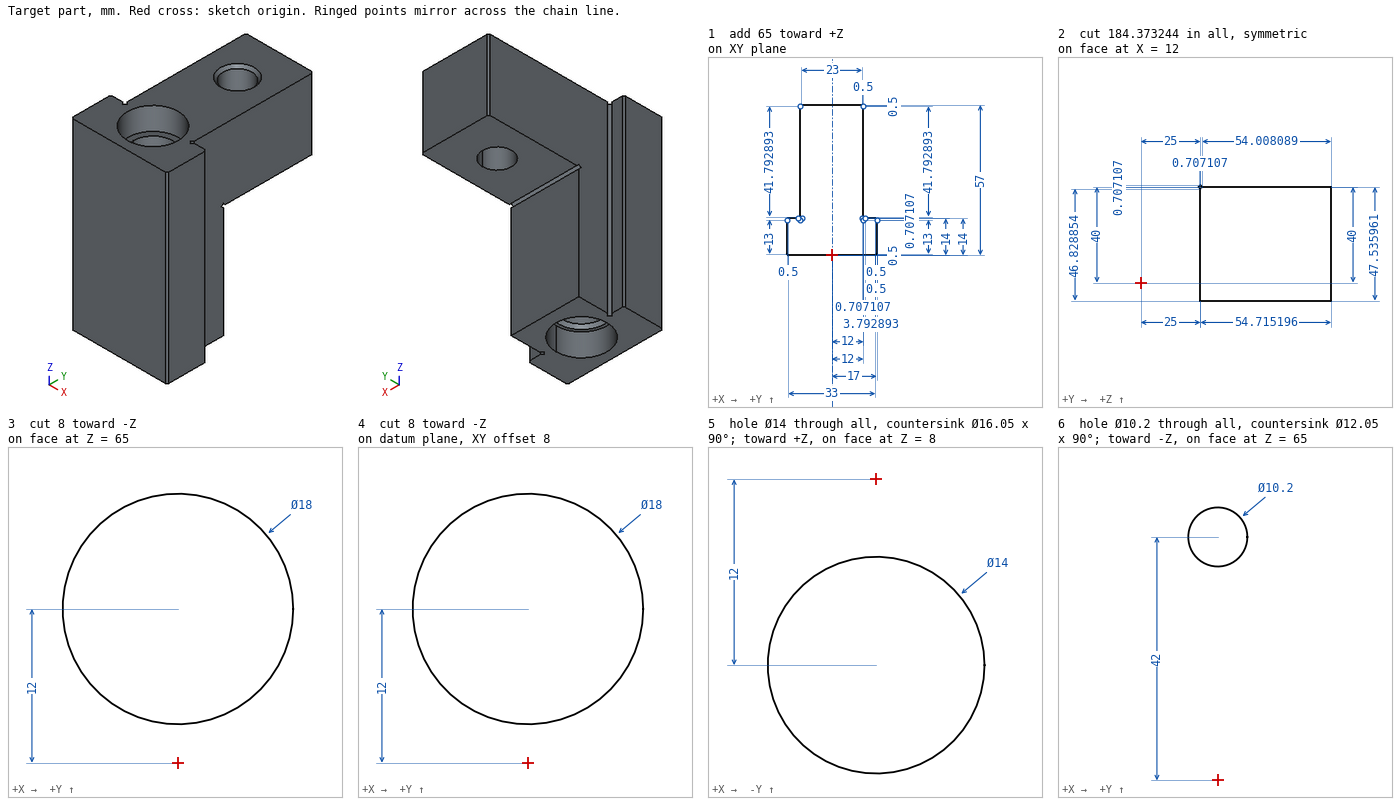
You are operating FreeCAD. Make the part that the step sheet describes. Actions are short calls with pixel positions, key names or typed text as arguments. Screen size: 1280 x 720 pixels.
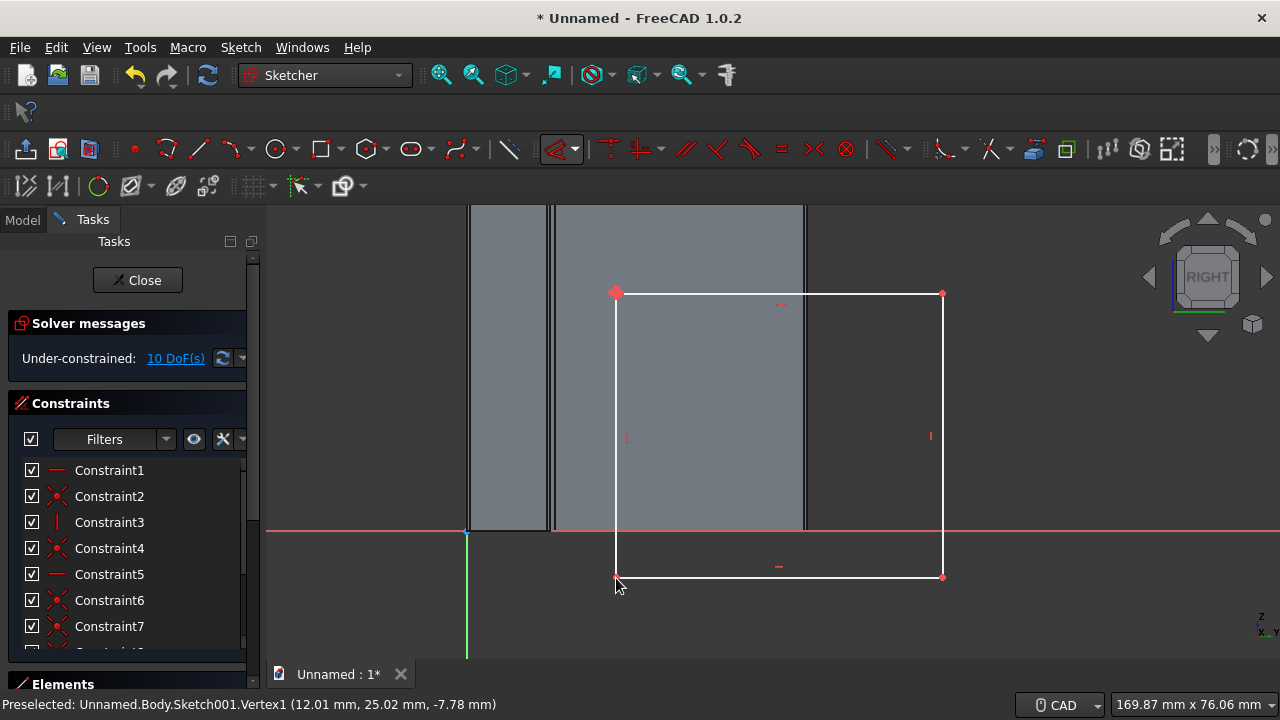
key(d)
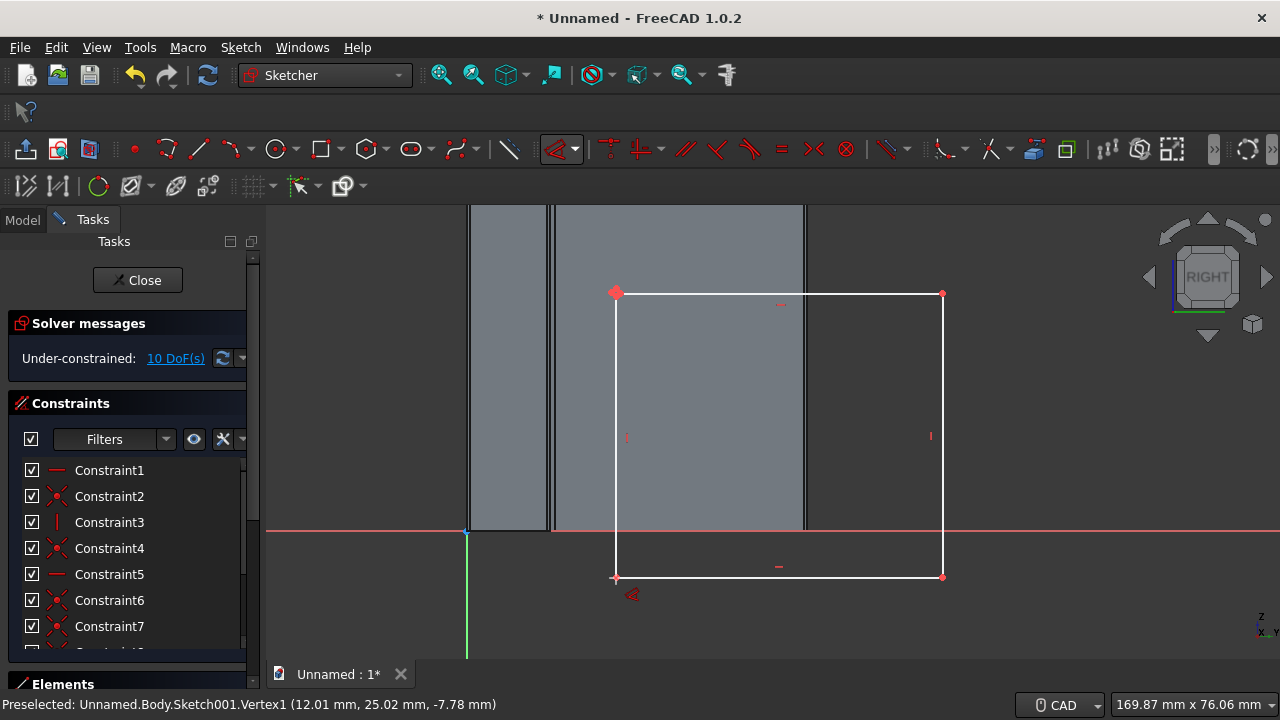
click(616, 578)
click(542, 612)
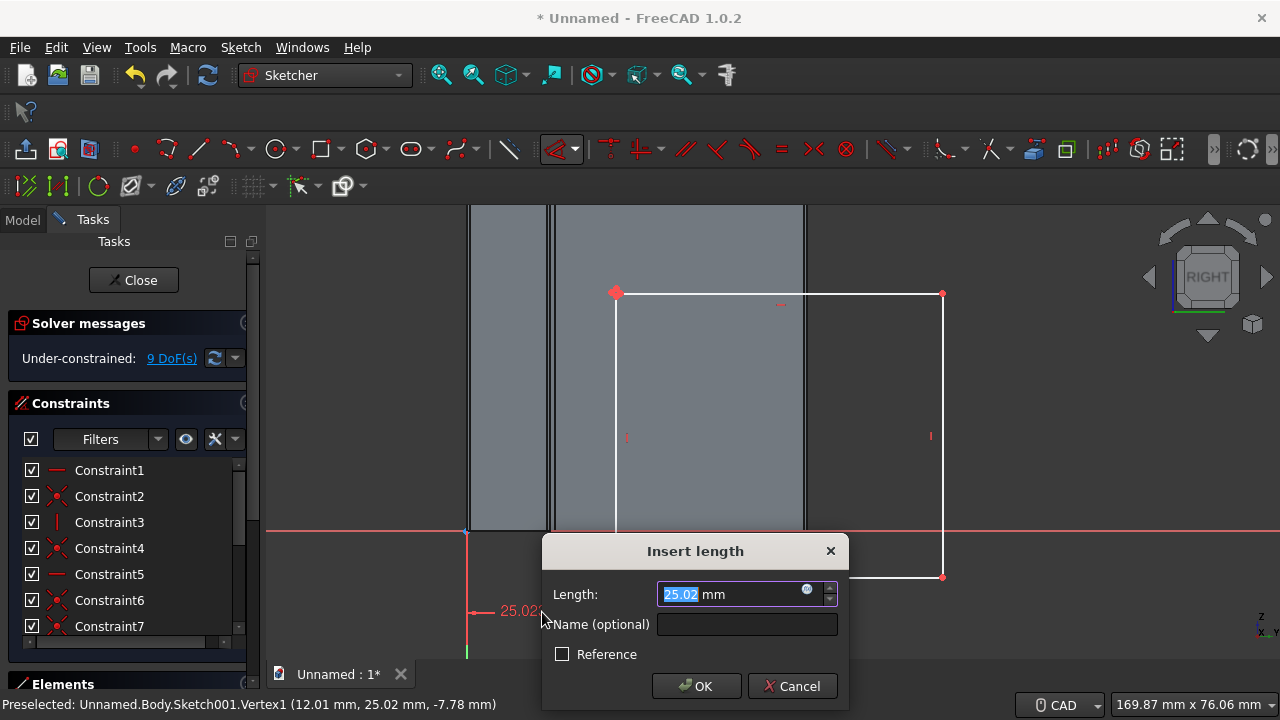
text(25)
key(Return)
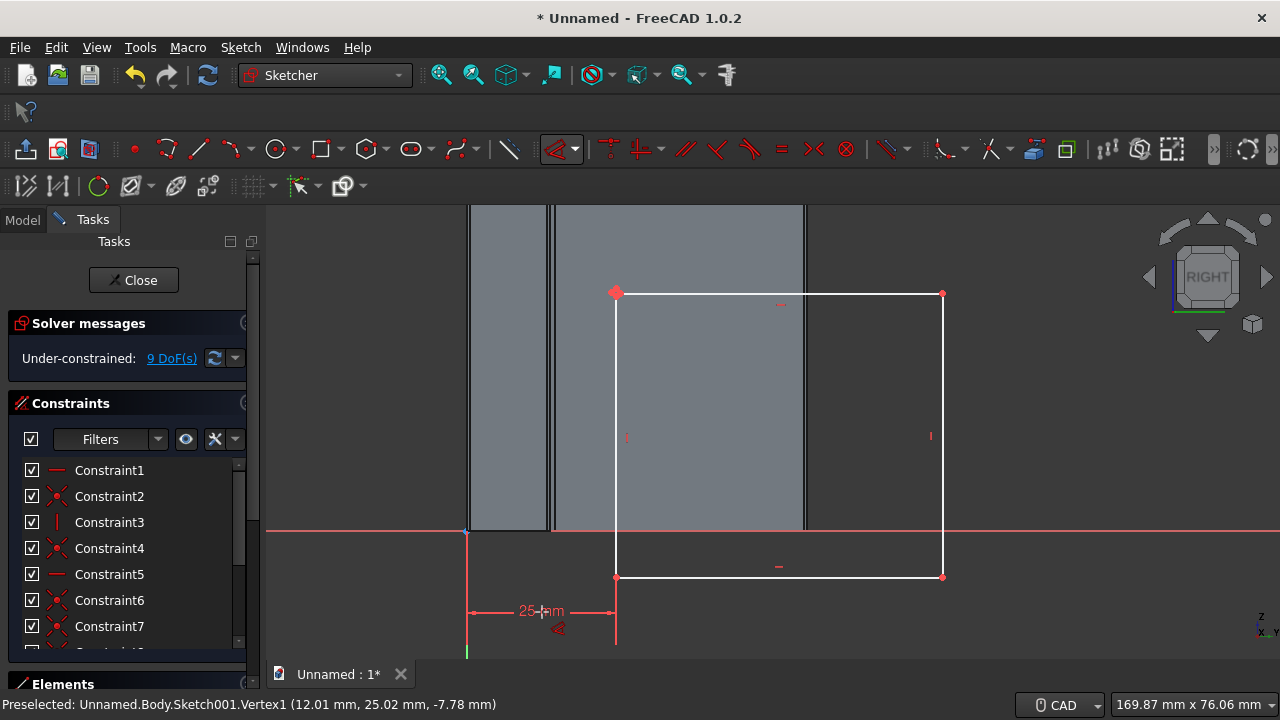
click(943, 294)
click(433, 412)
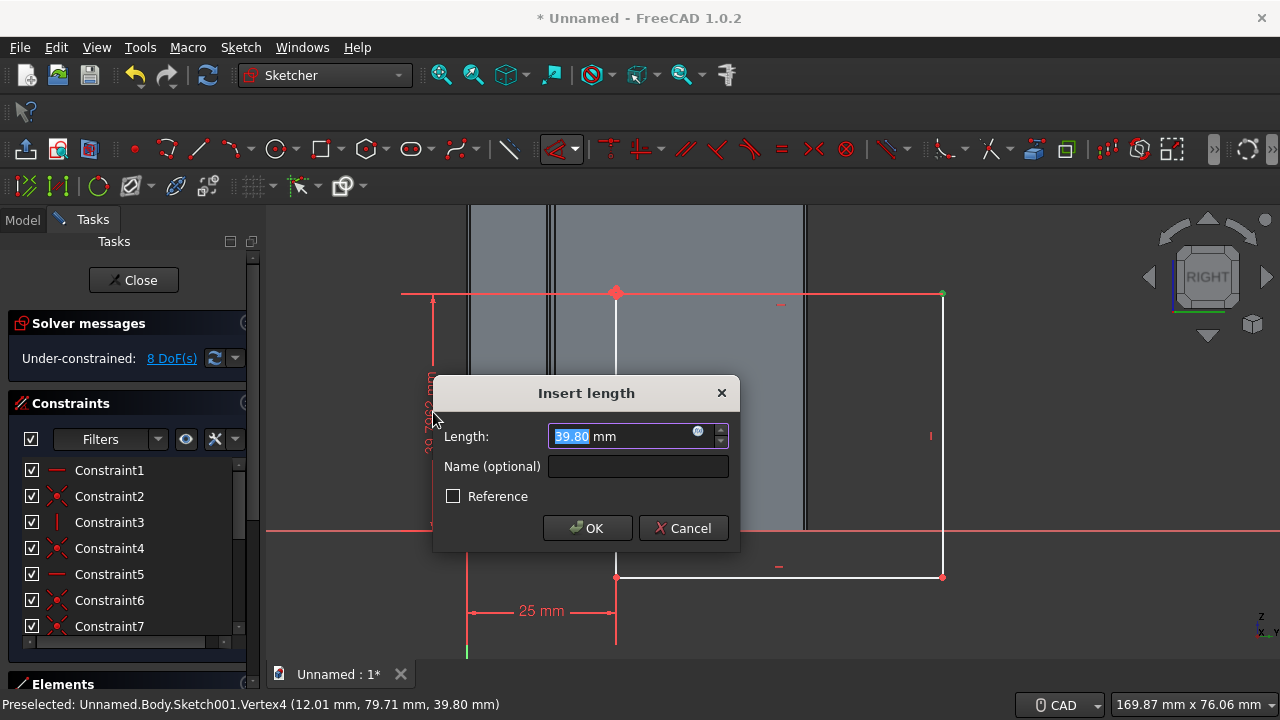
text(40)
key(Return)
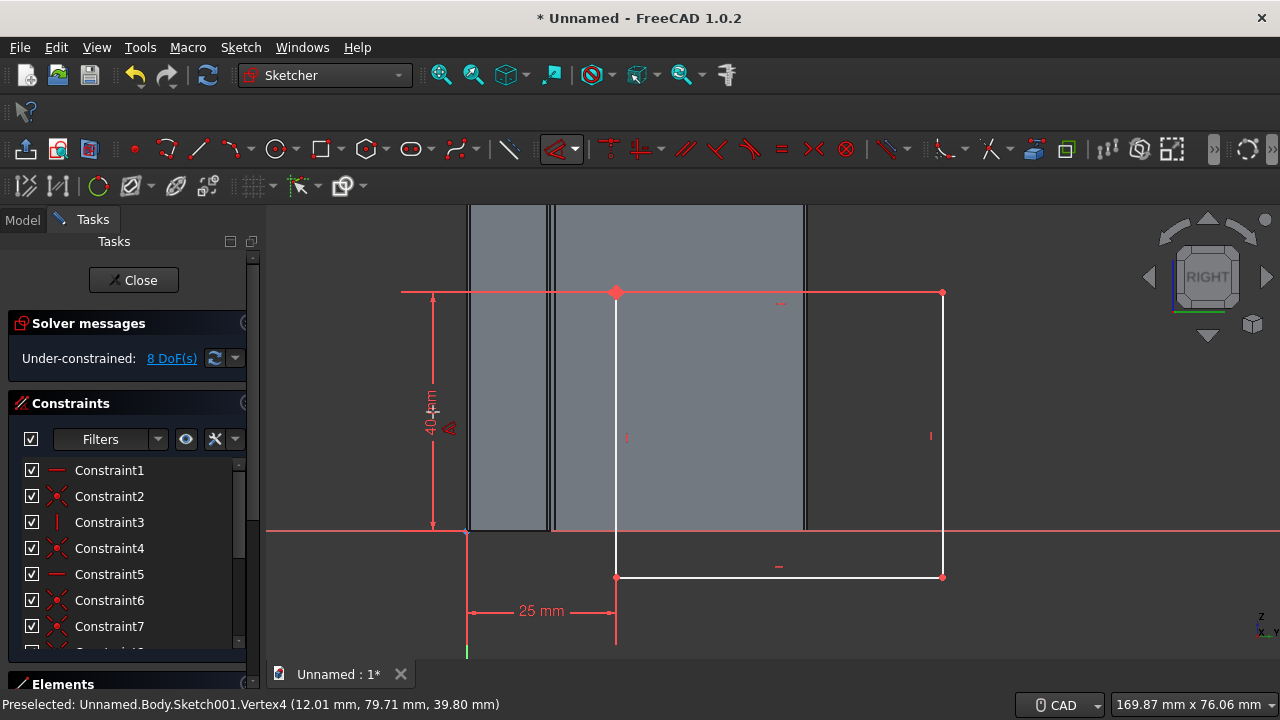
scroll(616, 288, up, 4)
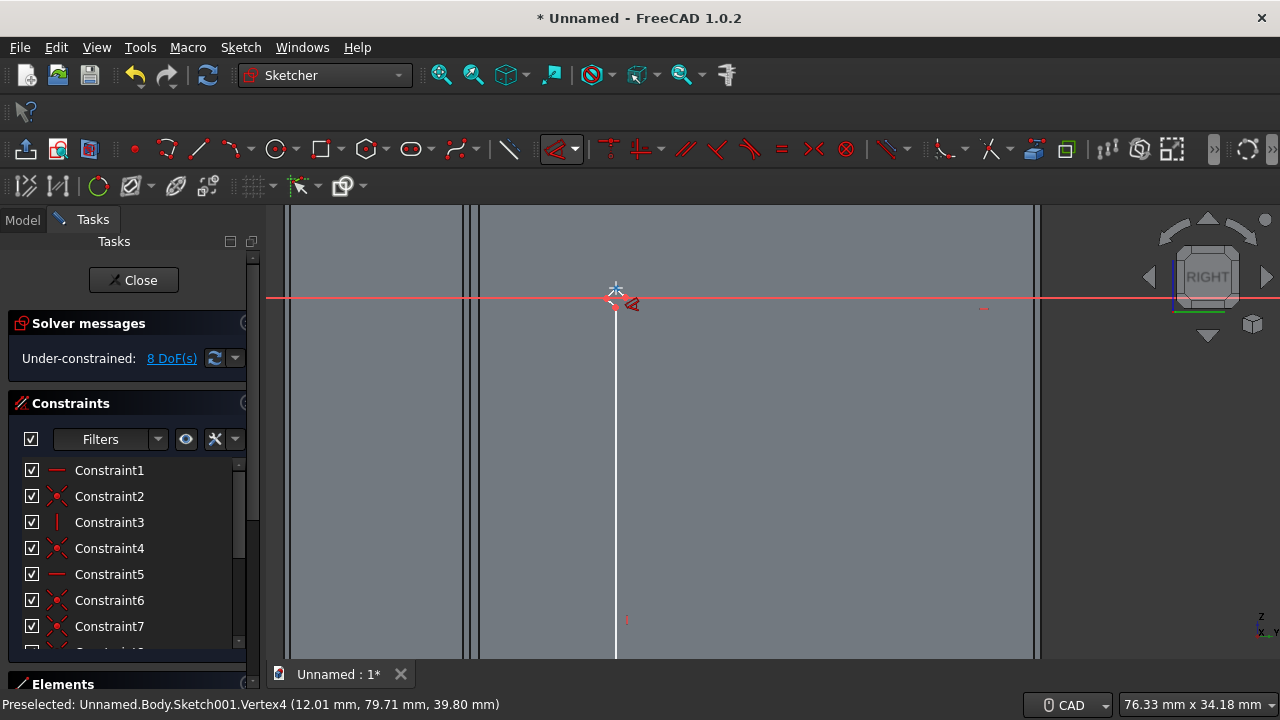
click(616, 289)
click(455, 255)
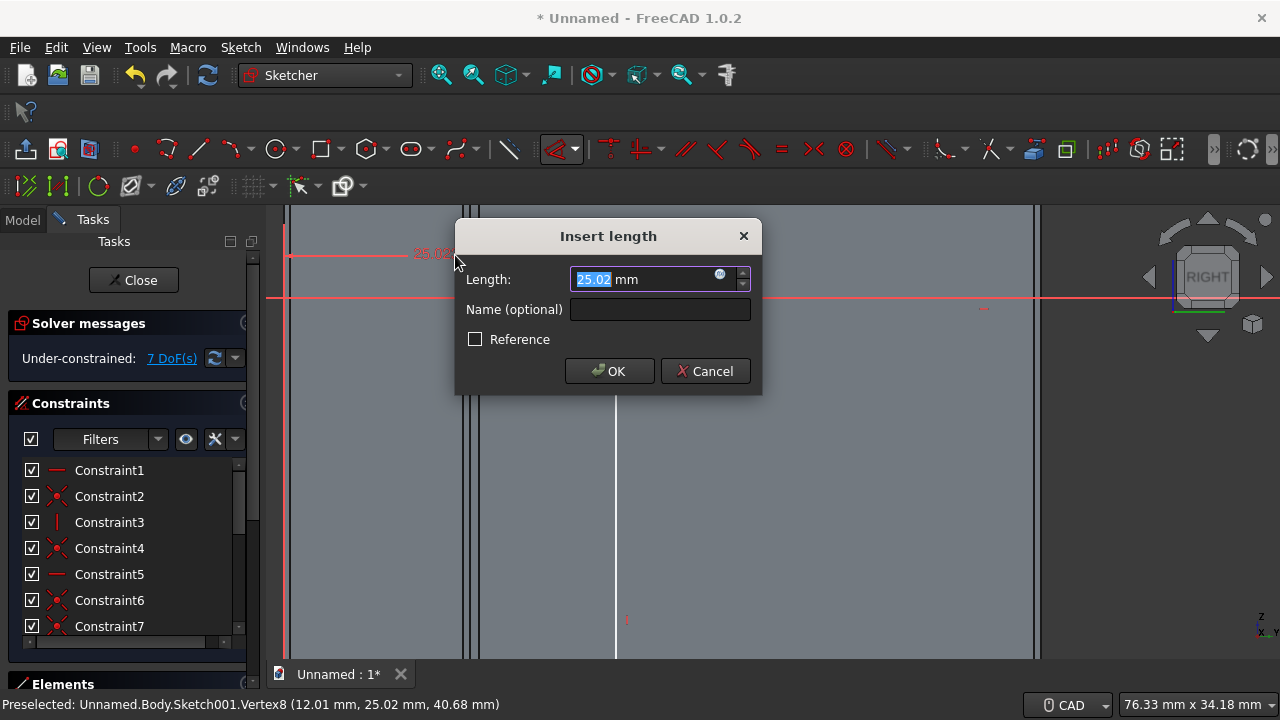
text(25)
key(Return)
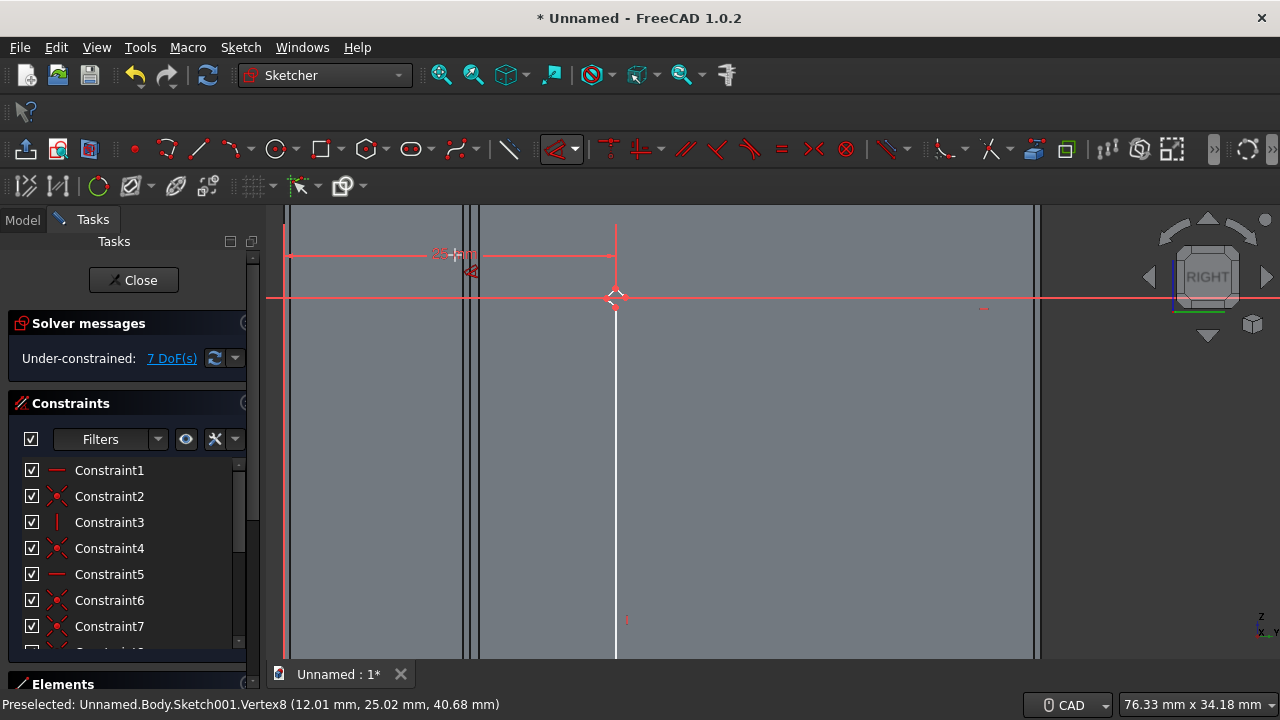
click(606, 298)
click(640, 465)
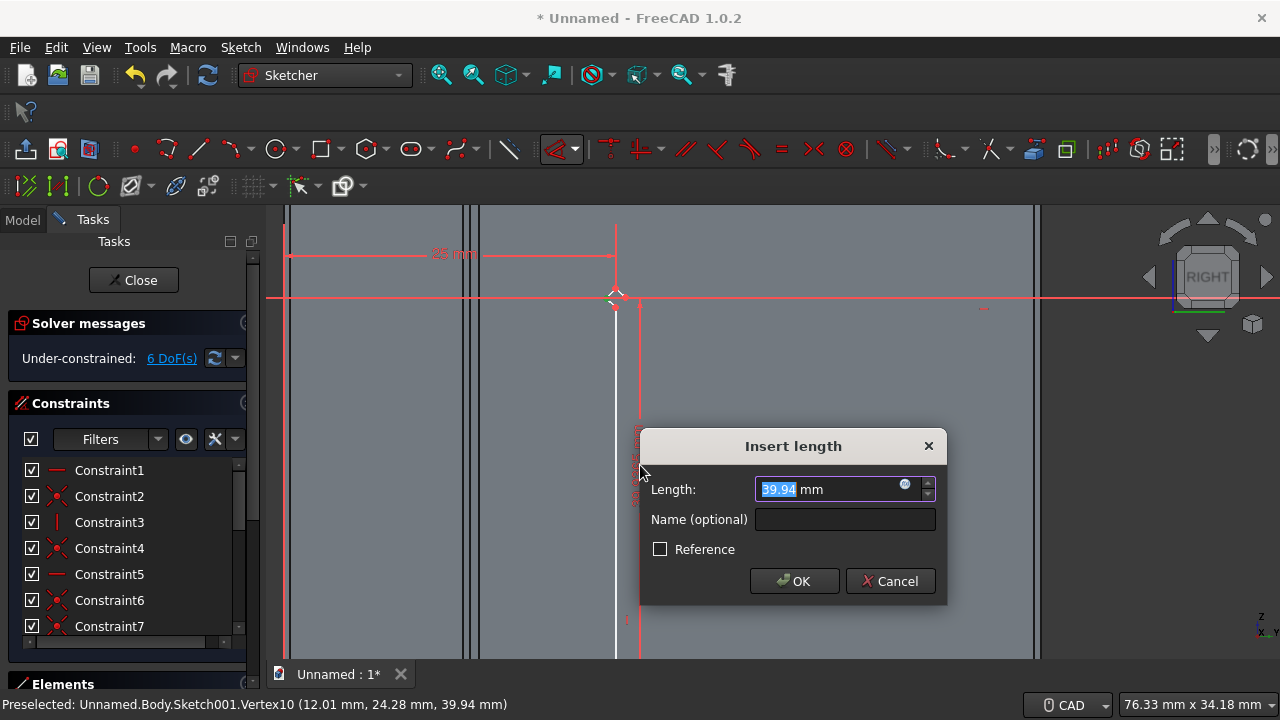
text(40)
key(Return)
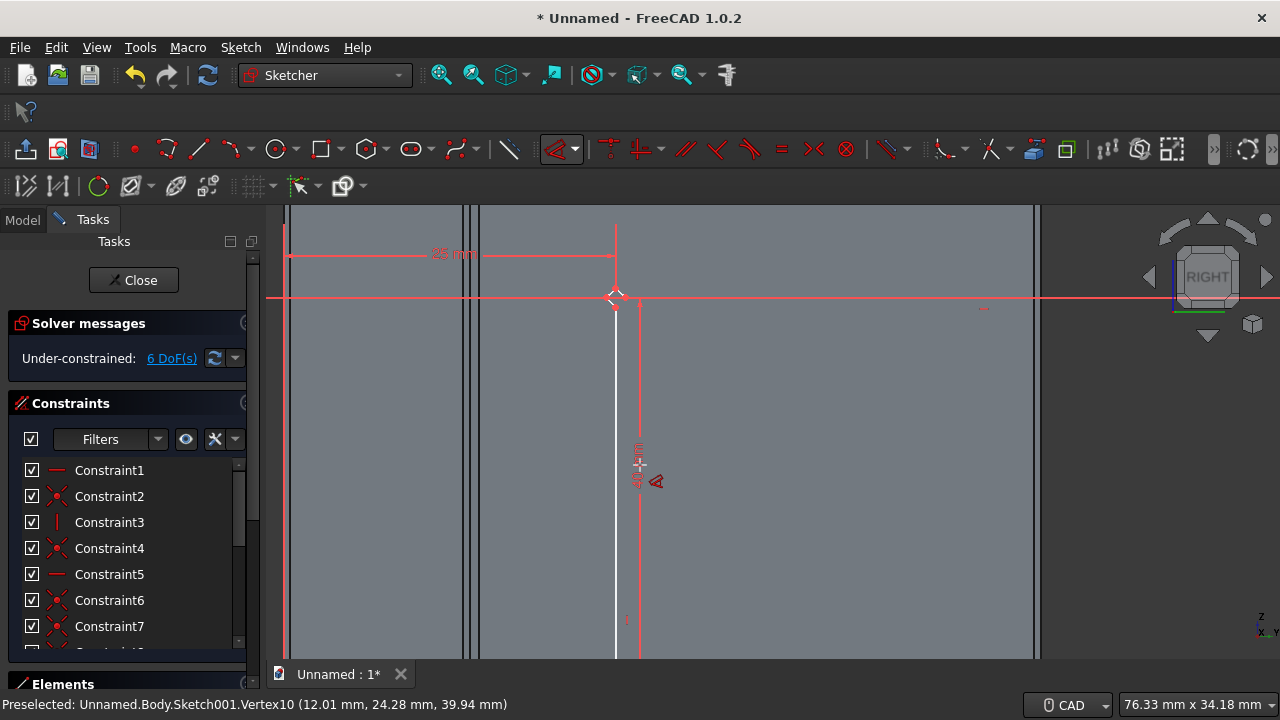
scroll(616, 288, down, 4)